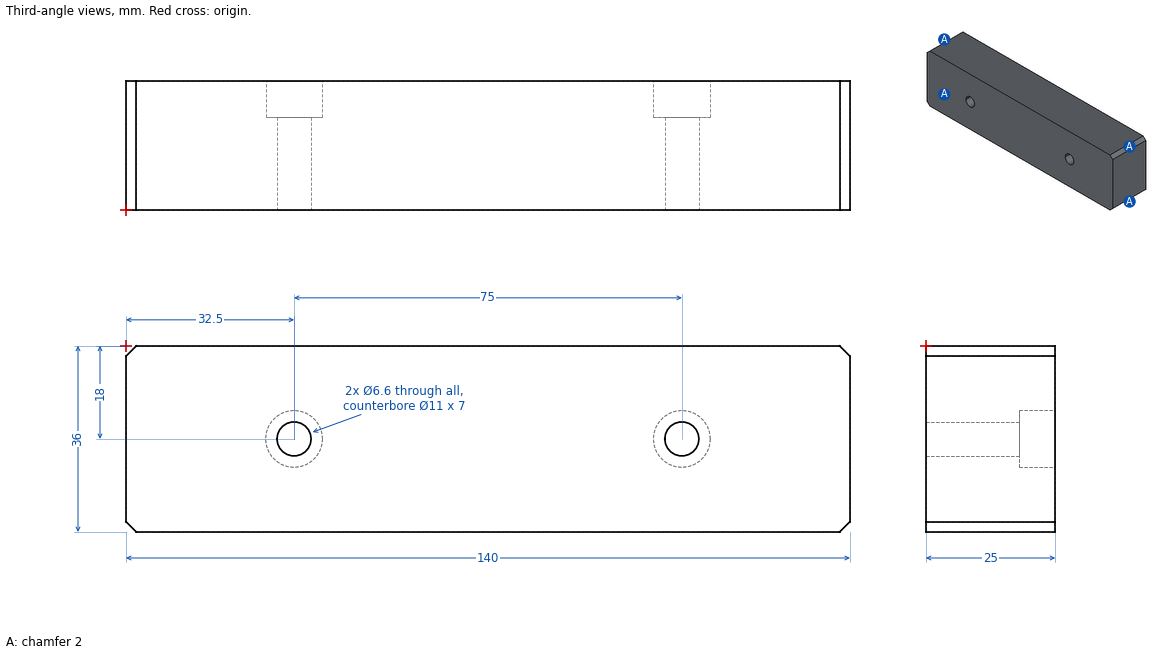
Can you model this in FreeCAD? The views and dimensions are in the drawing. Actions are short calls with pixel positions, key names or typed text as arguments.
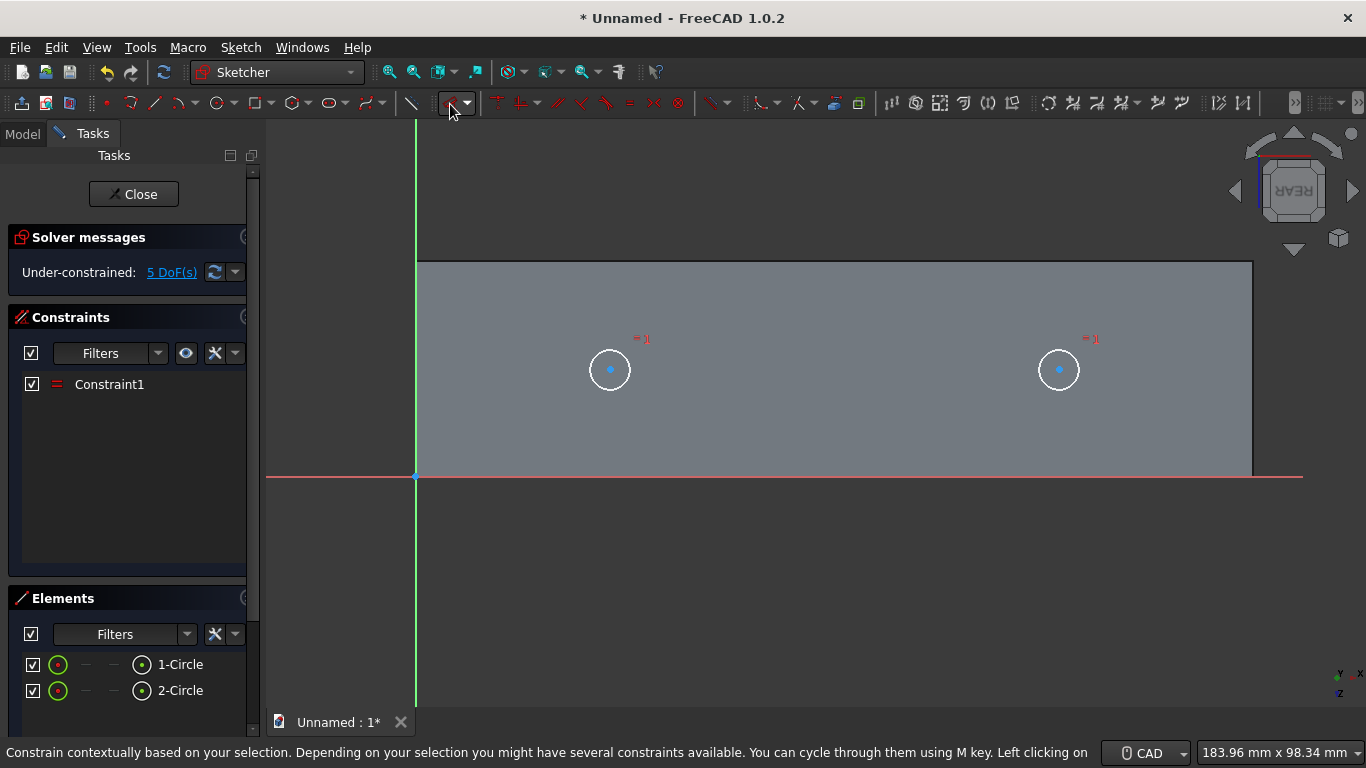
click(624, 356)
click(647, 333)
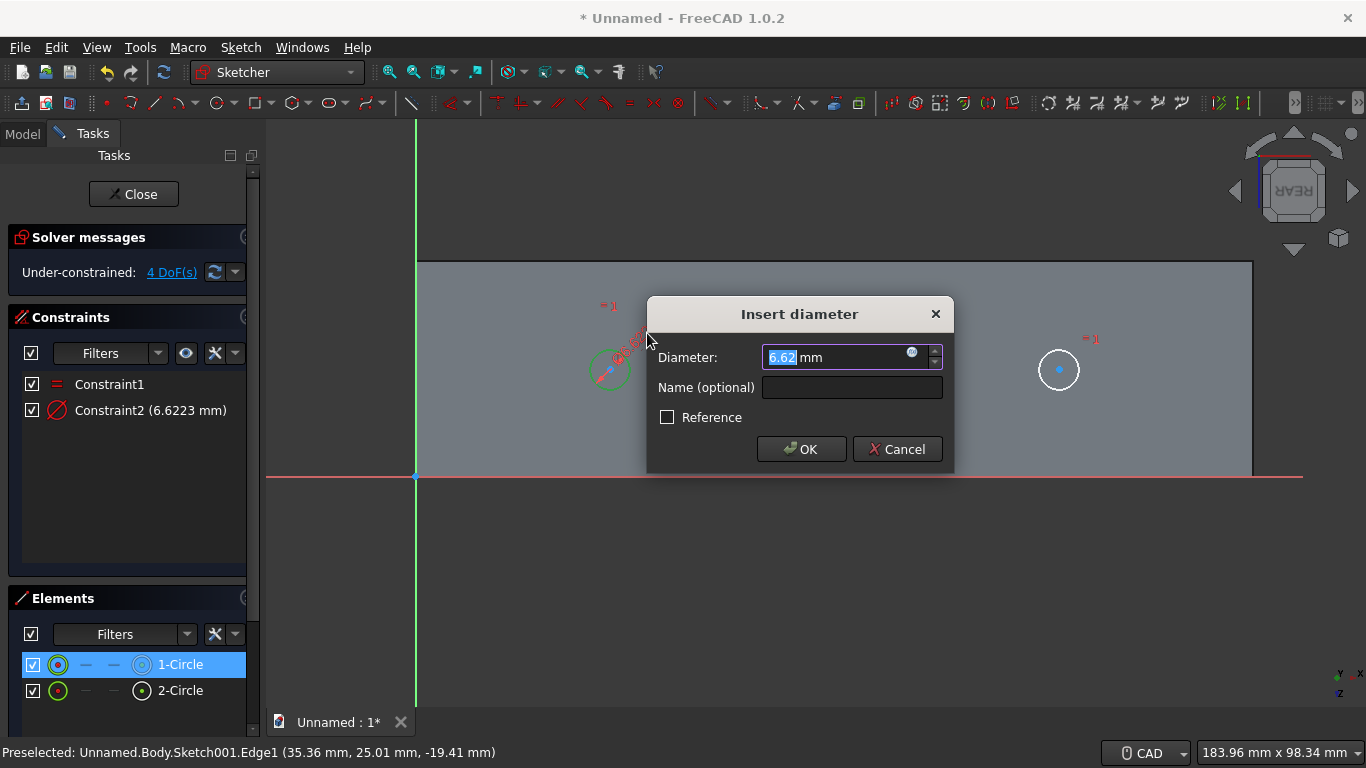
text(6.6)
key(Return)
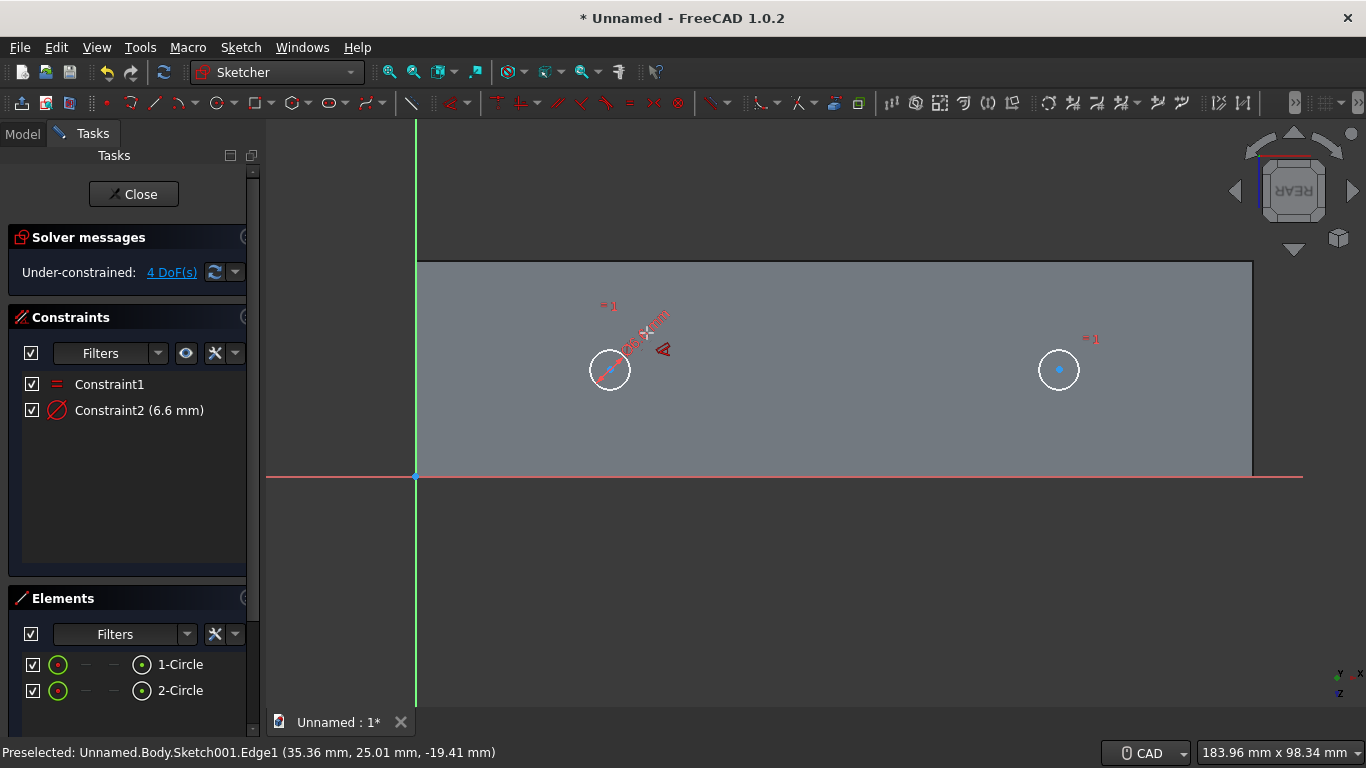
click(610, 370)
click(382, 423)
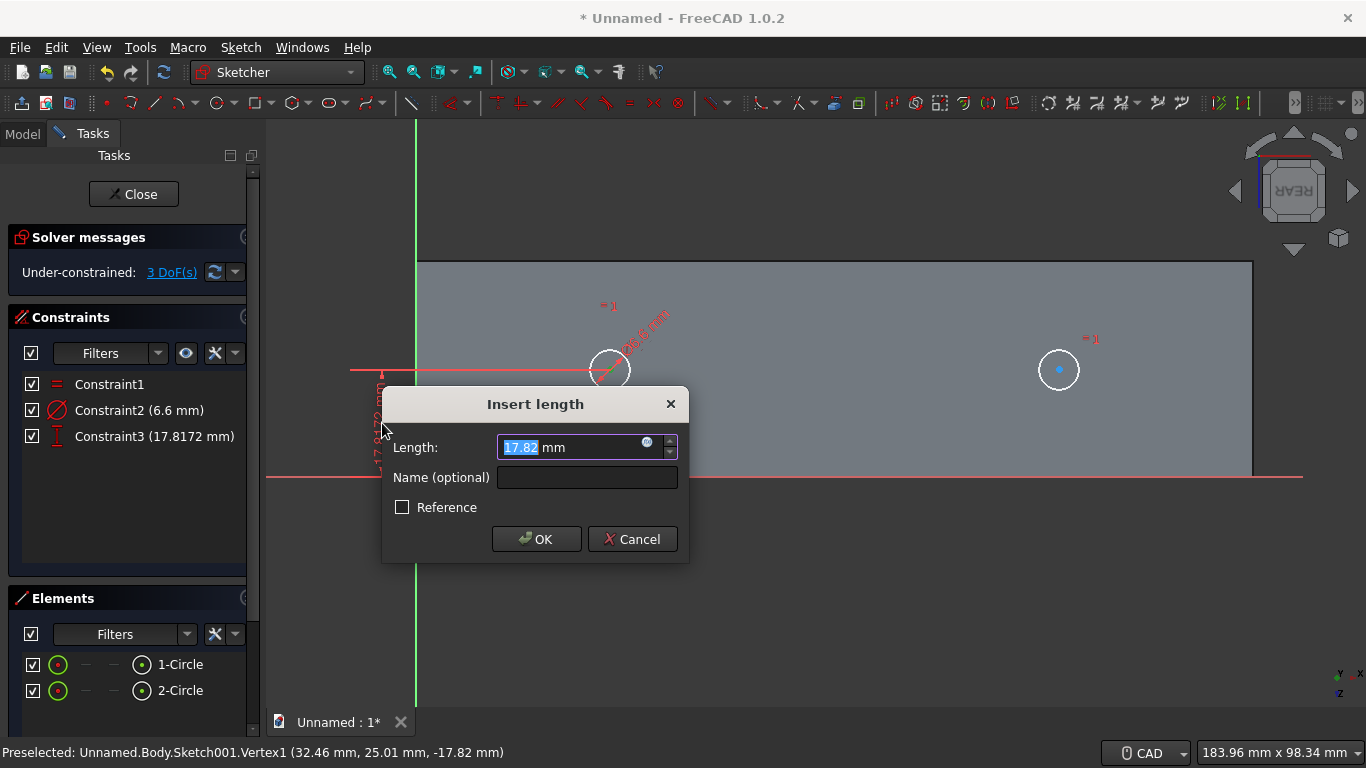
text(18)
key(Return)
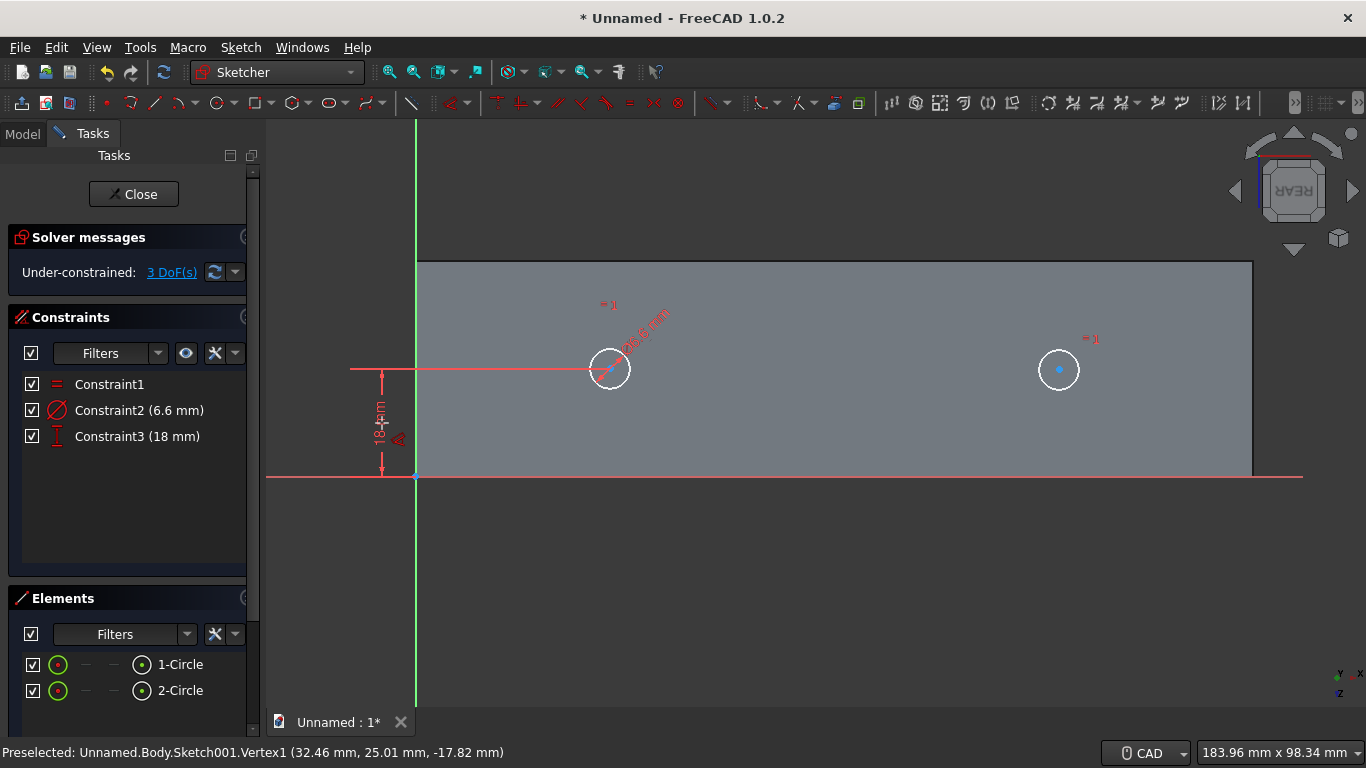
click(1059, 370)
click(382, 399)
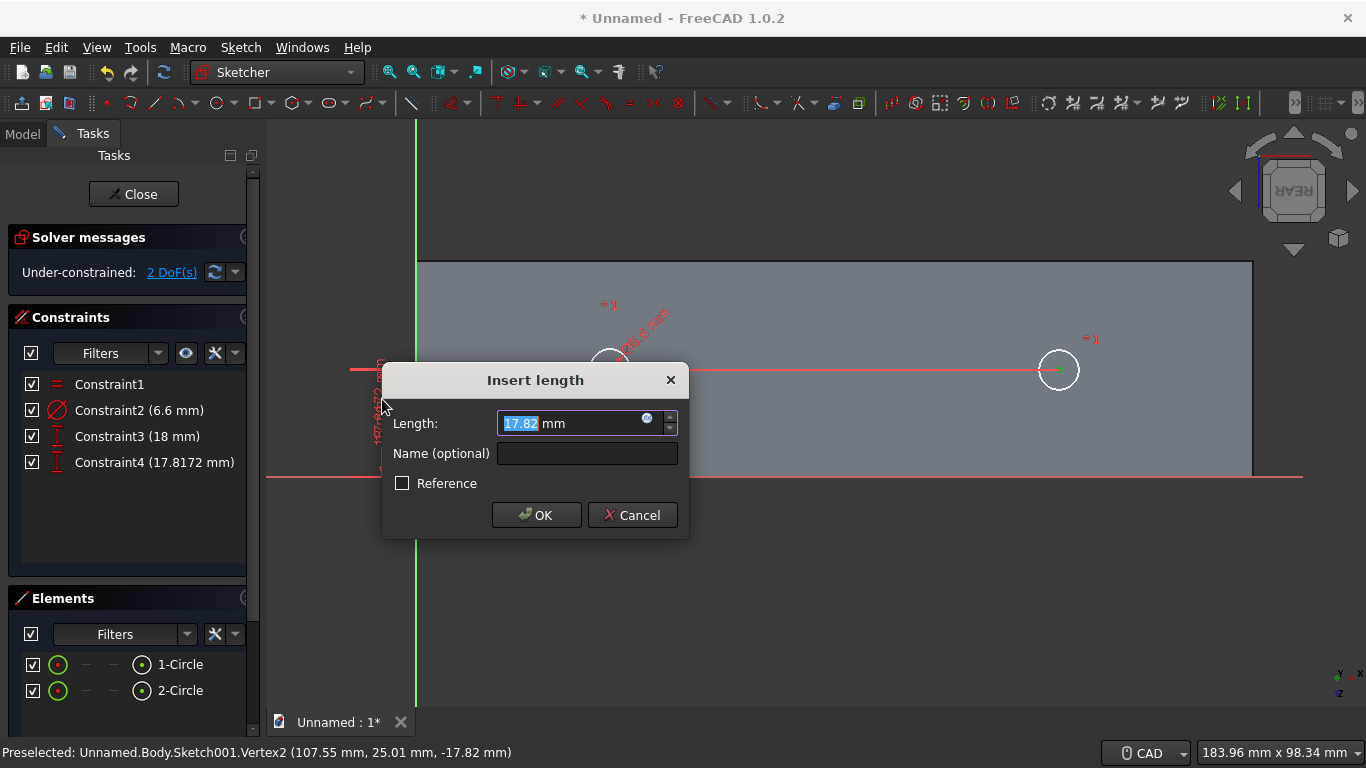
text(18)
key(Return)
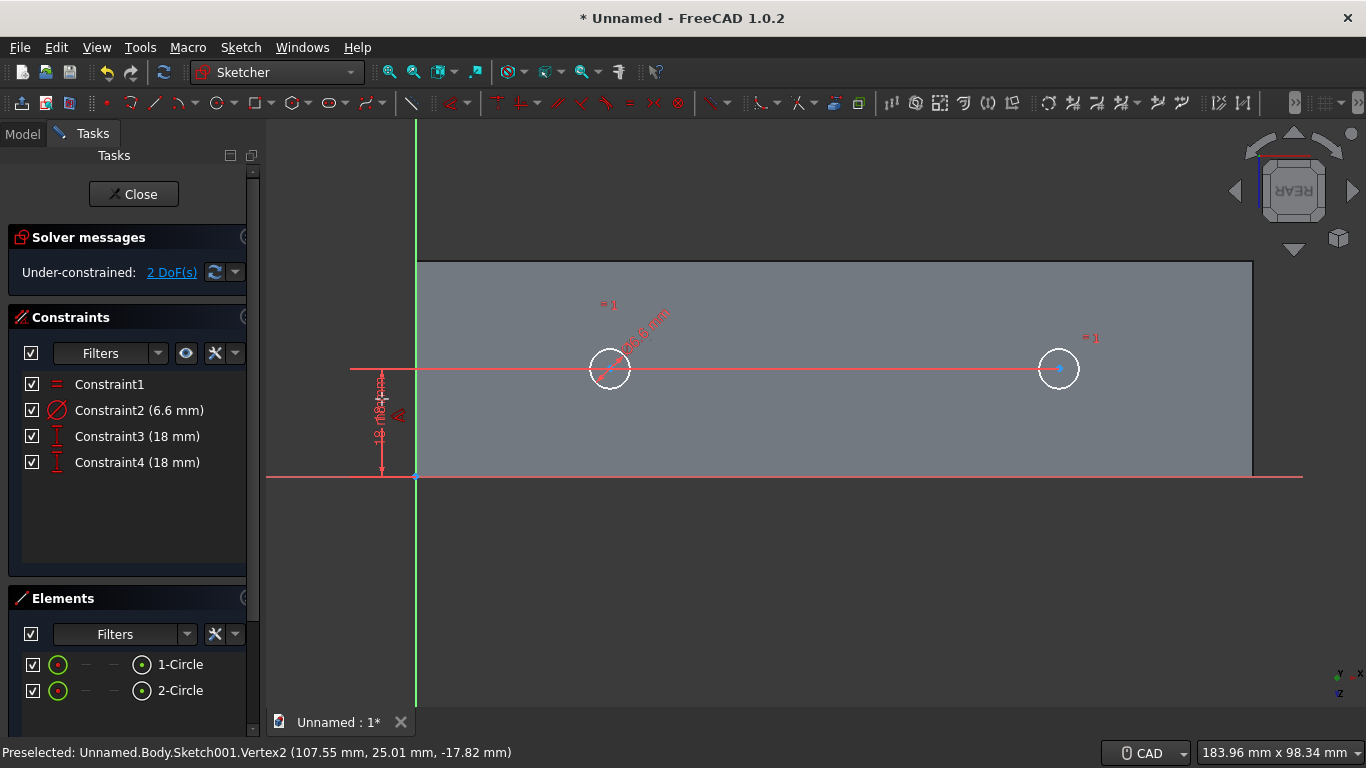
click(610, 369)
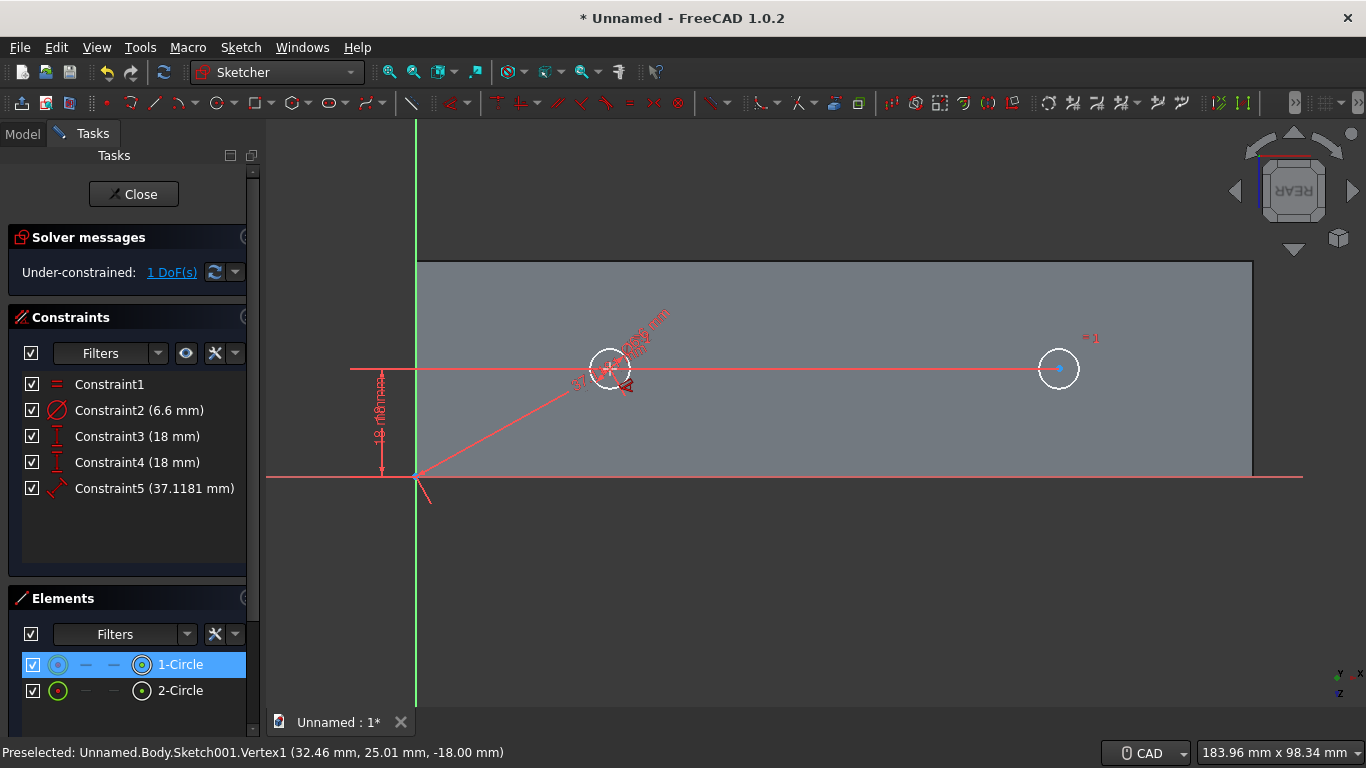
click(1059, 369)
click(835, 335)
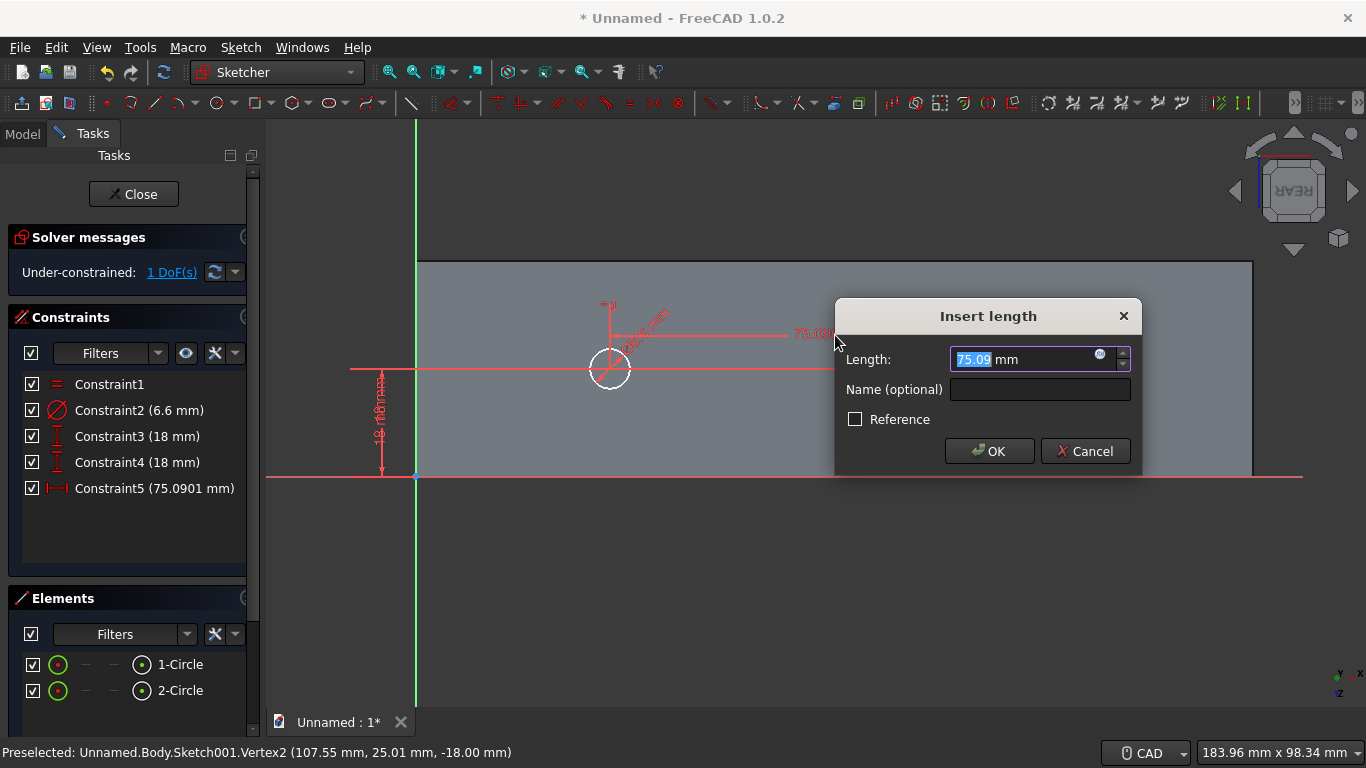
text(75)
key(Return)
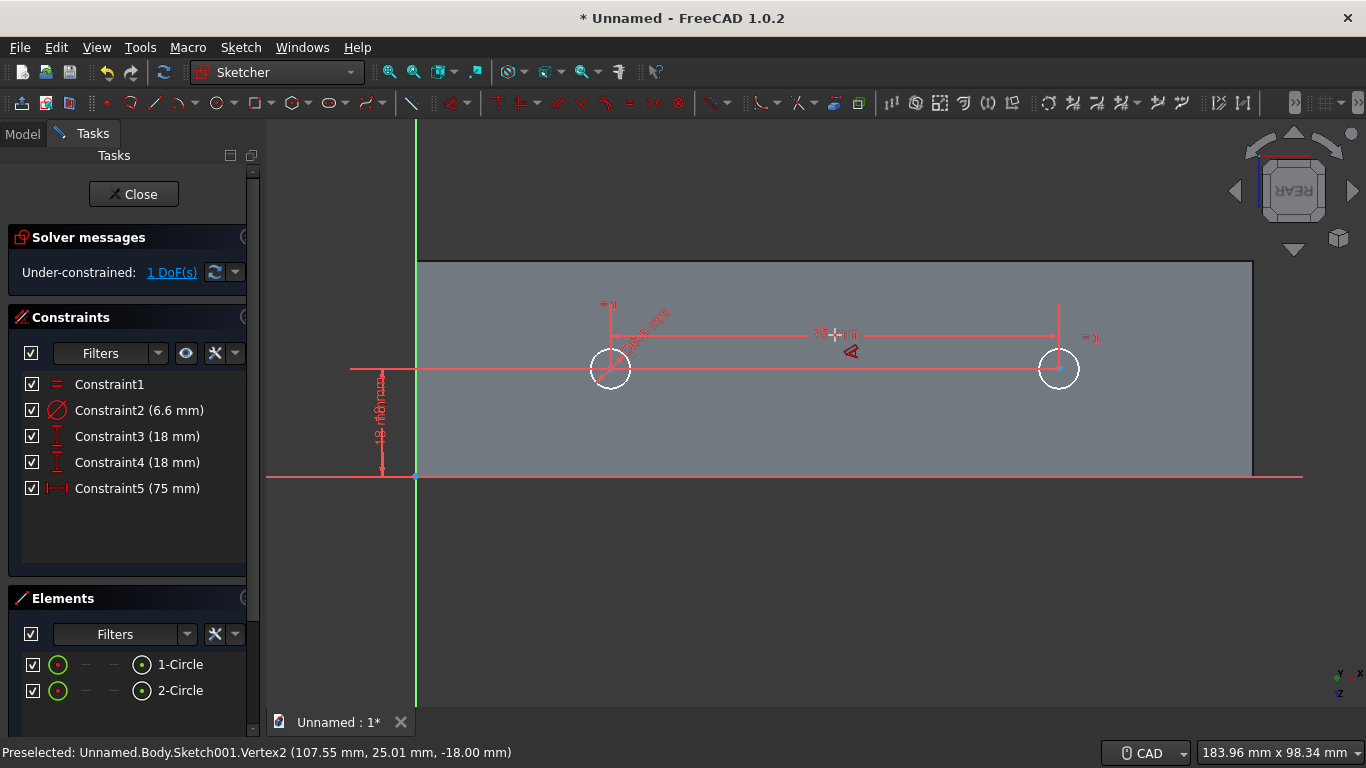
click(611, 369)
click(513, 511)